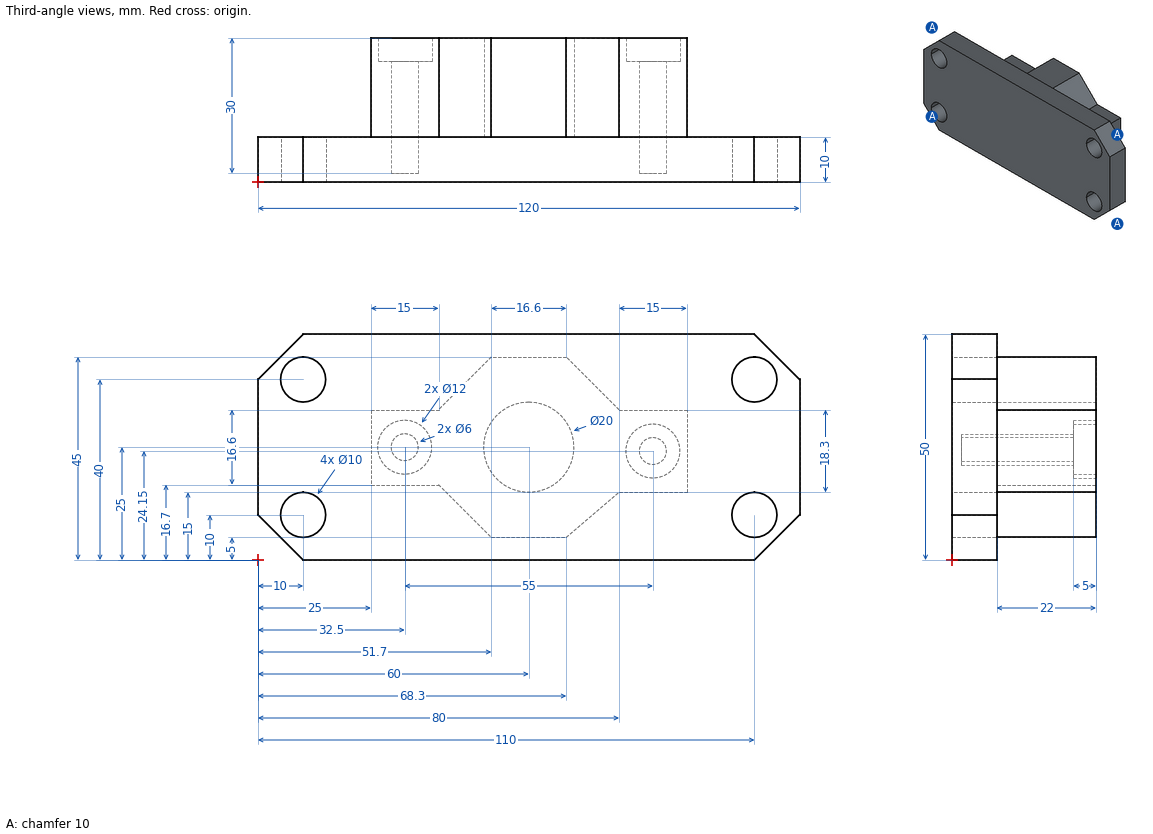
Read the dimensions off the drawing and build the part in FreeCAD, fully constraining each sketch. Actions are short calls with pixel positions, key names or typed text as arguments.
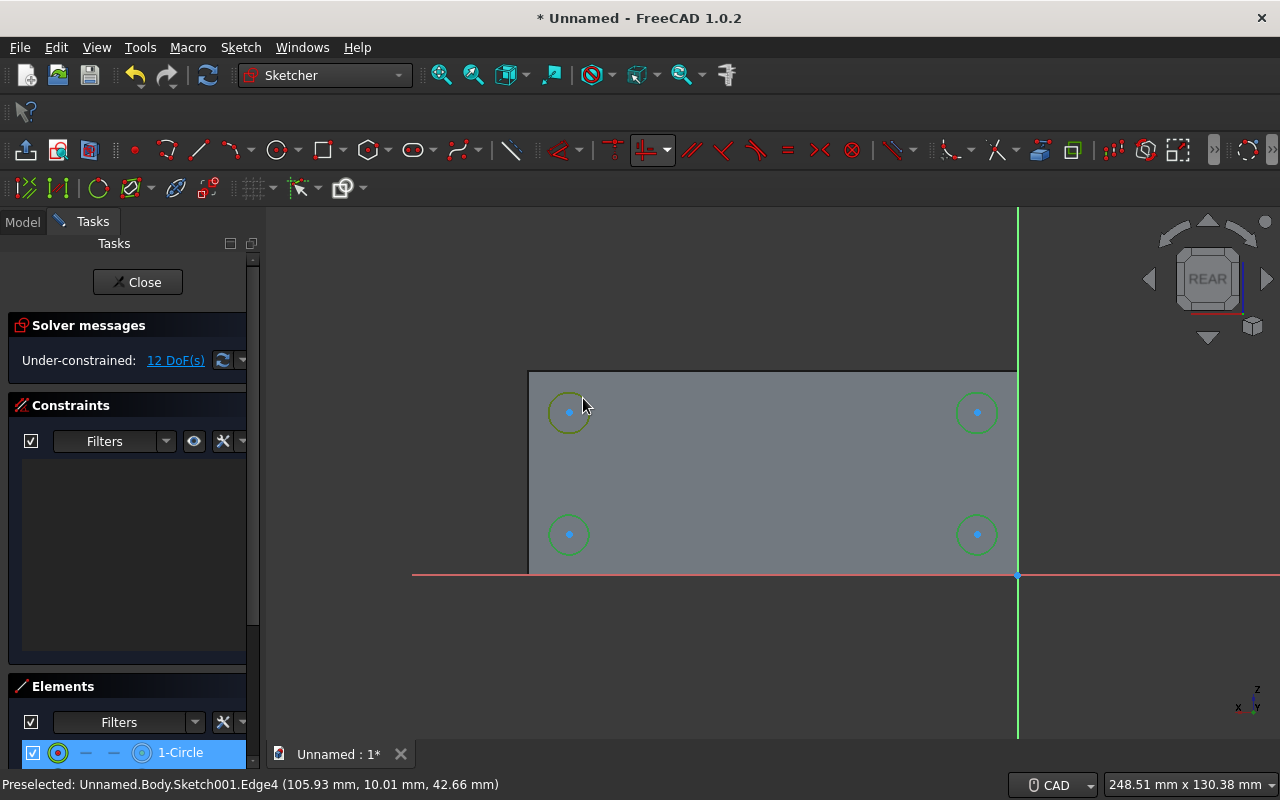
click(788, 150)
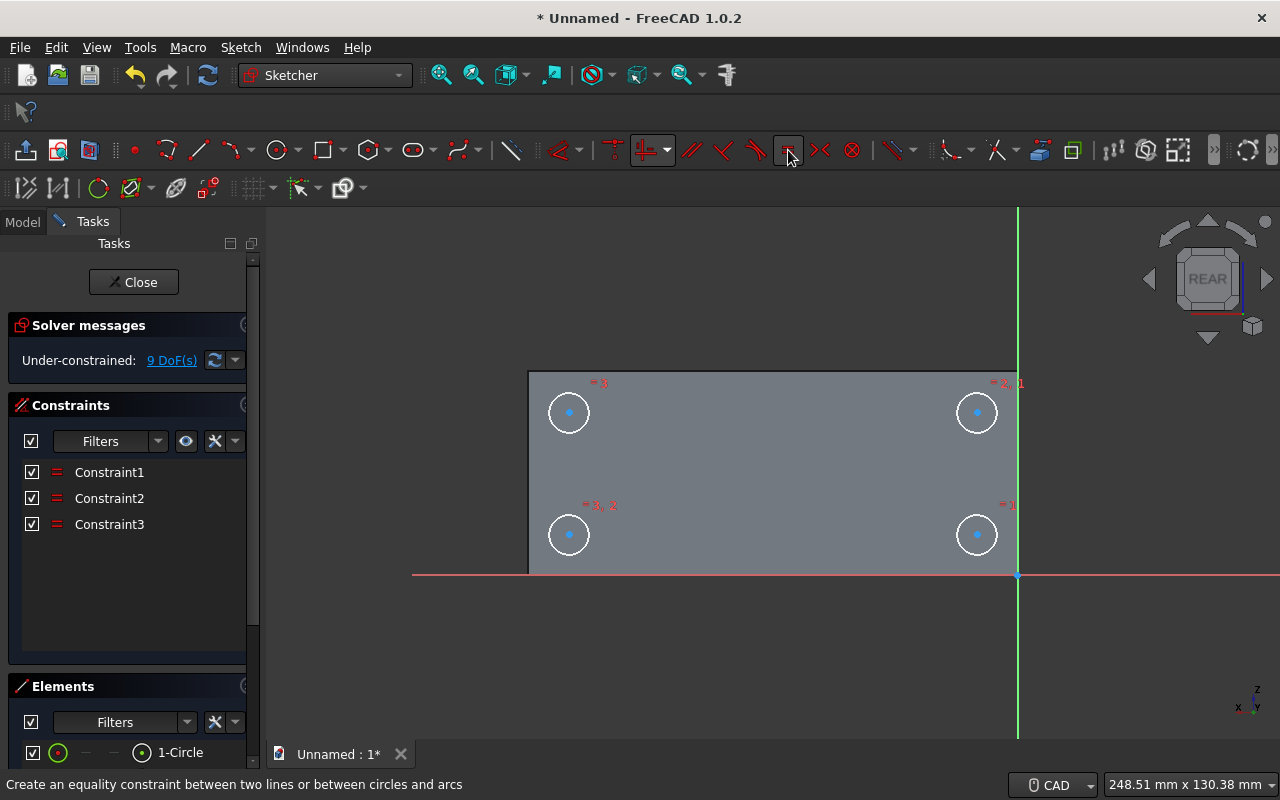
click(977, 535)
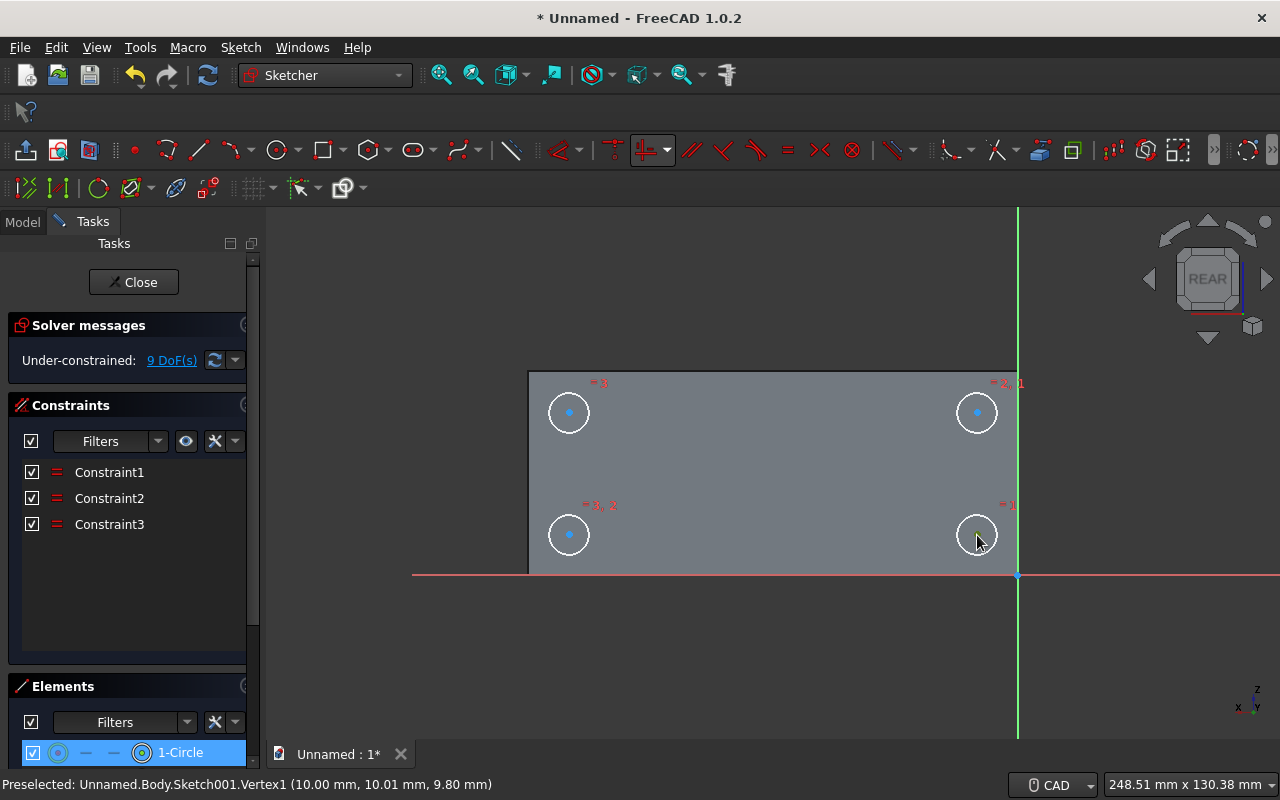
click(977, 413)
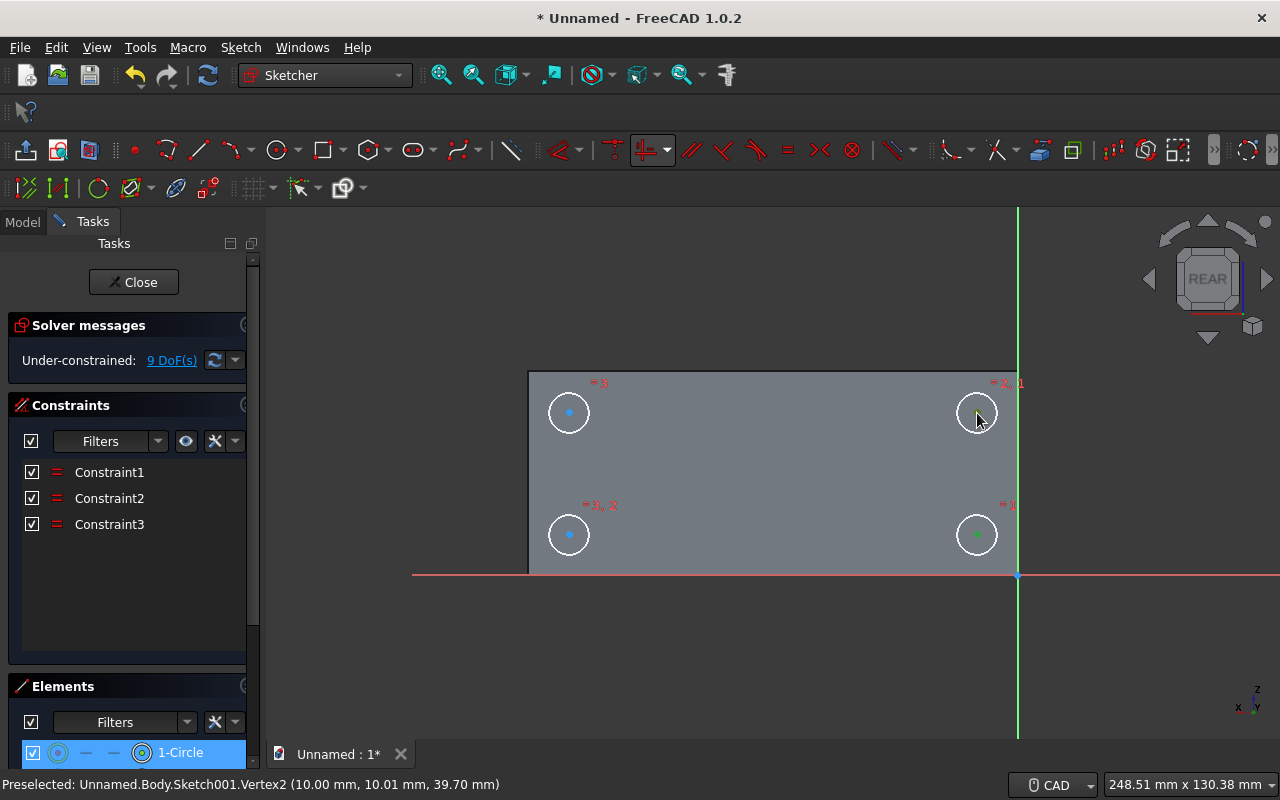
key(v)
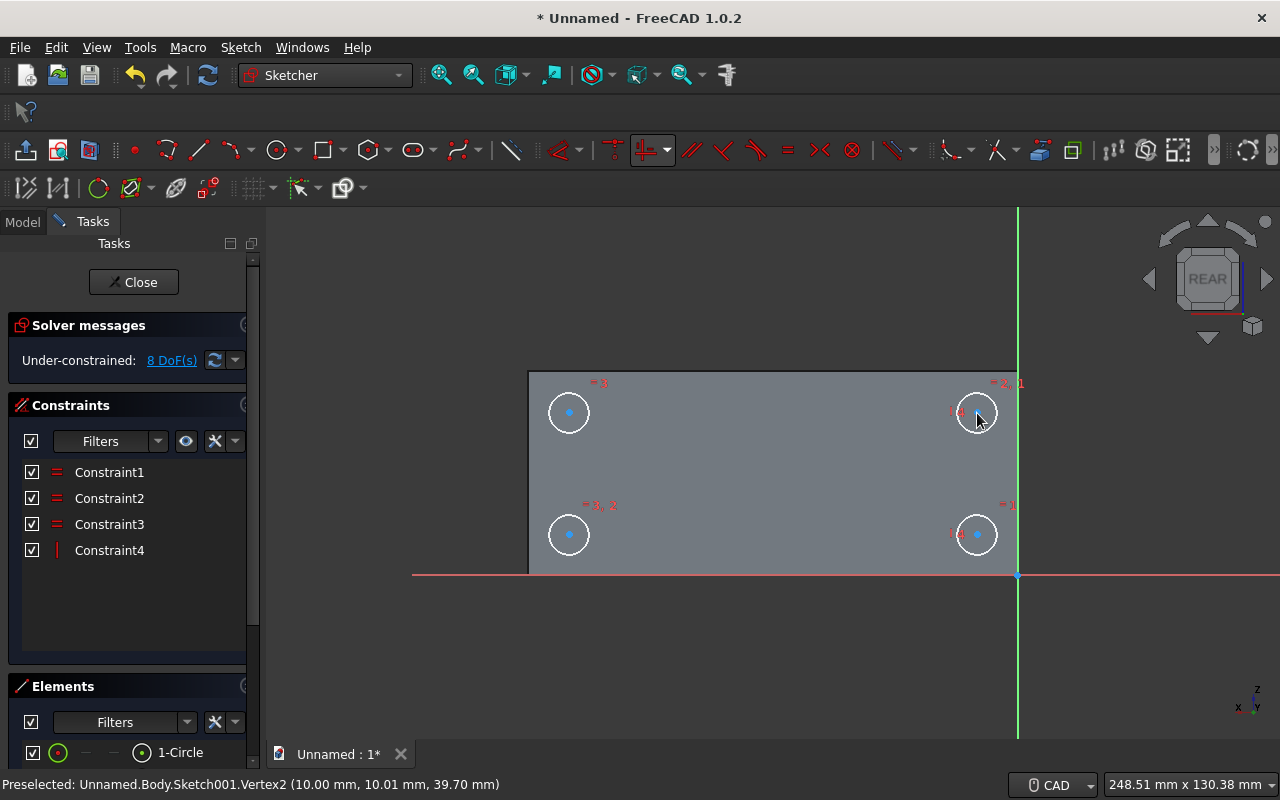
click(977, 535)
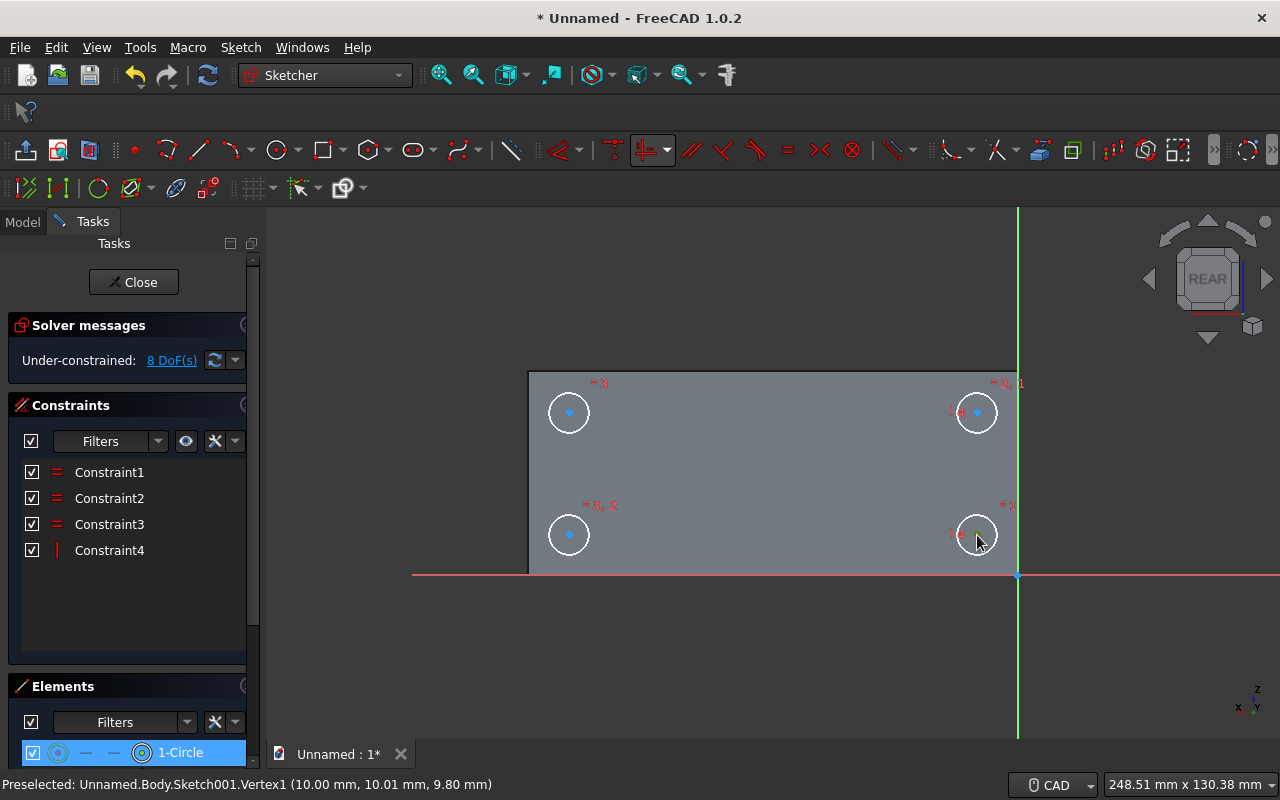
click(569, 535)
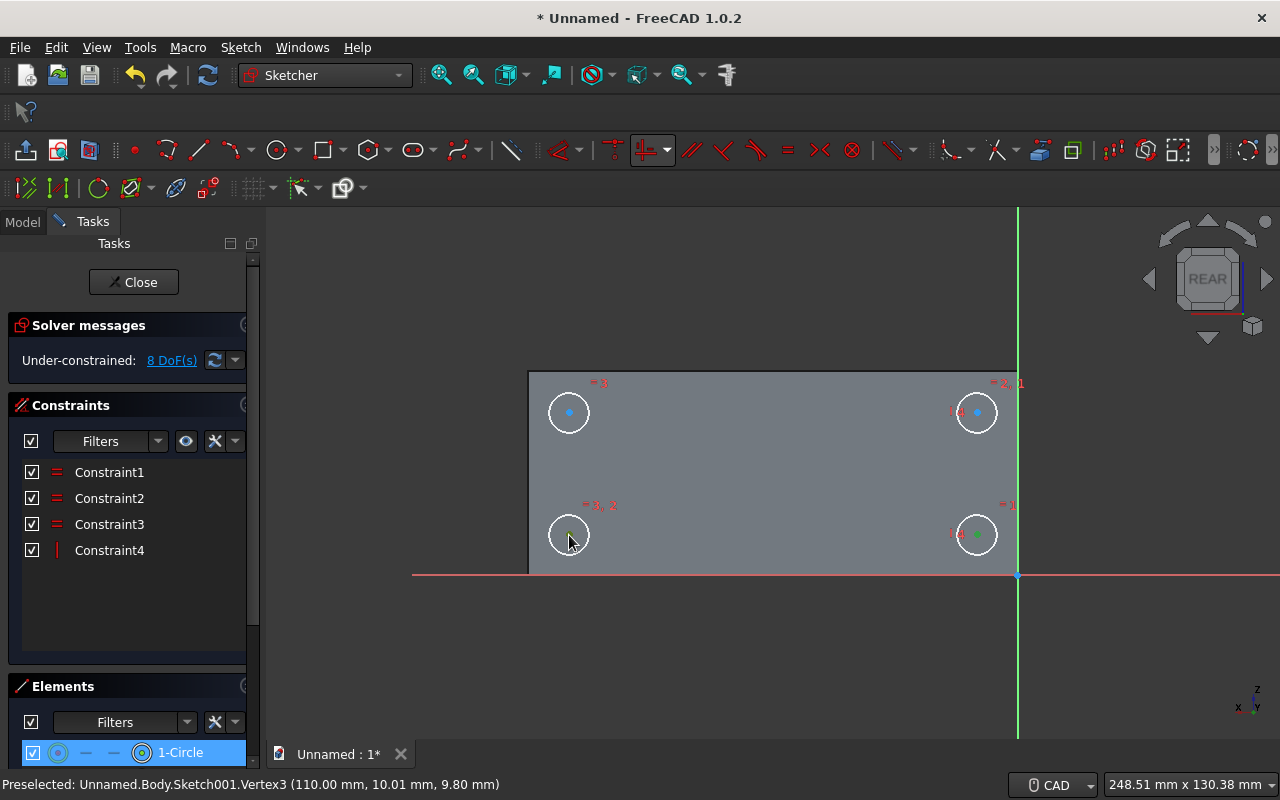
key(h)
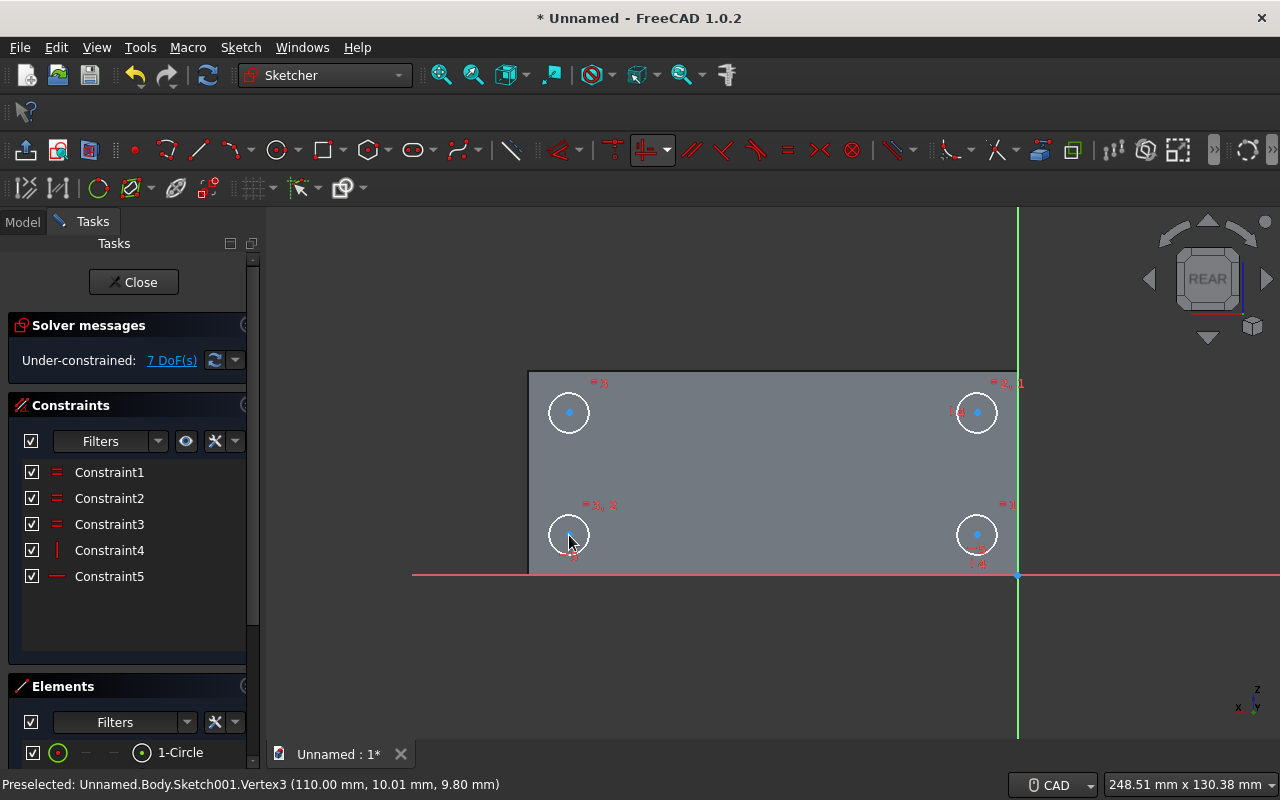
click(569, 535)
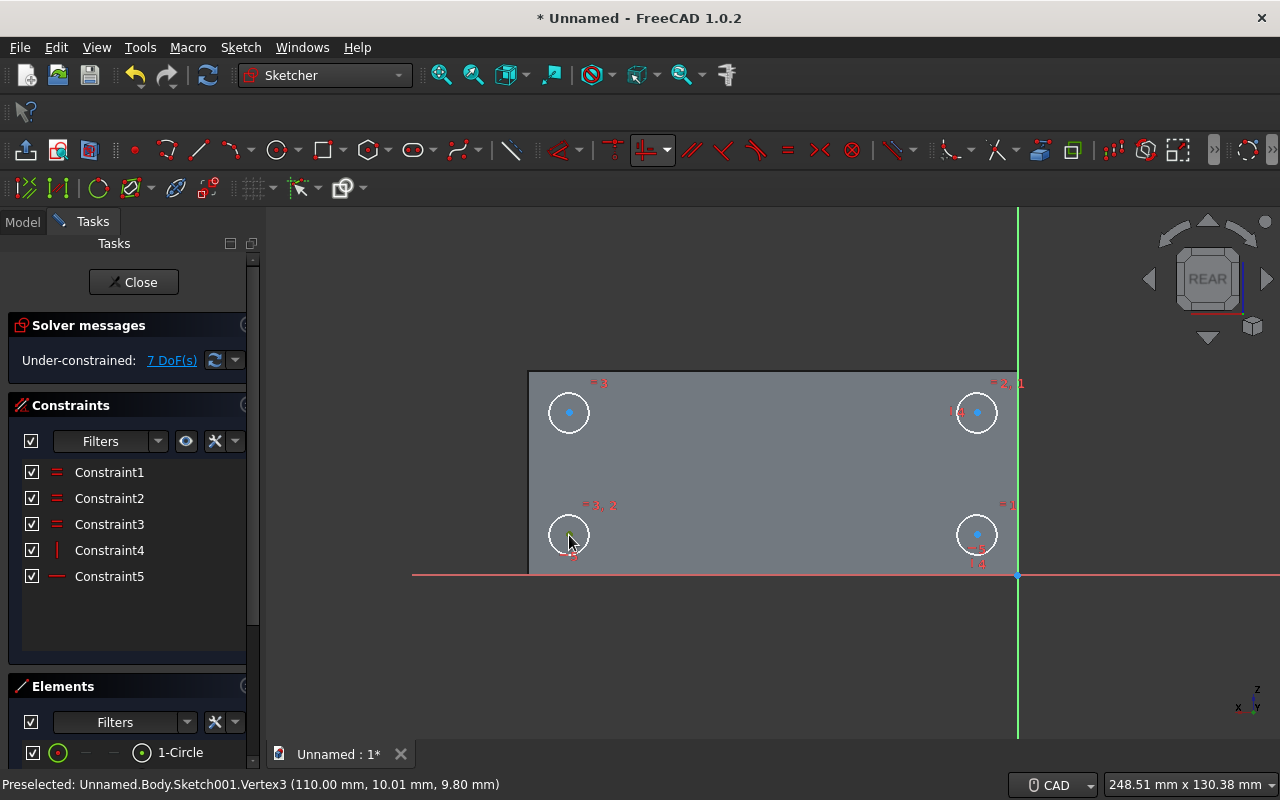
click(569, 413)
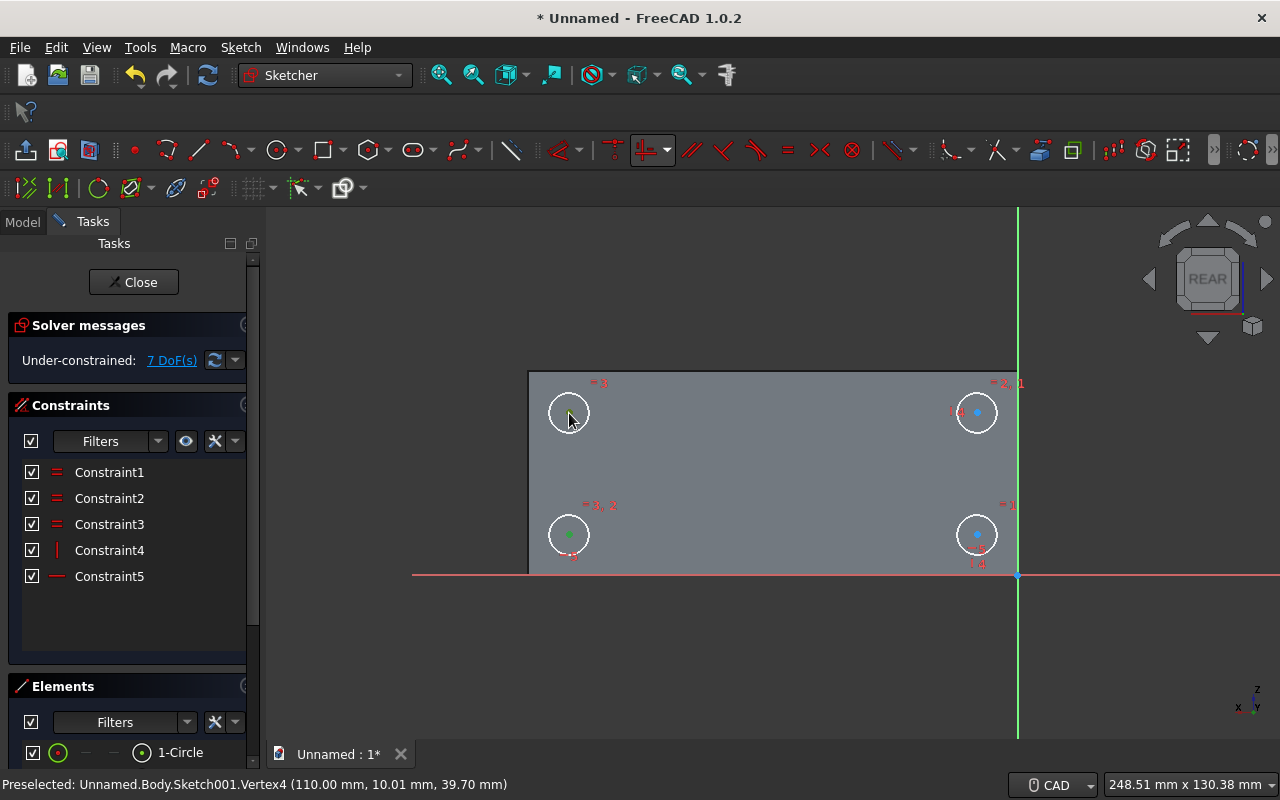
click(670, 150)